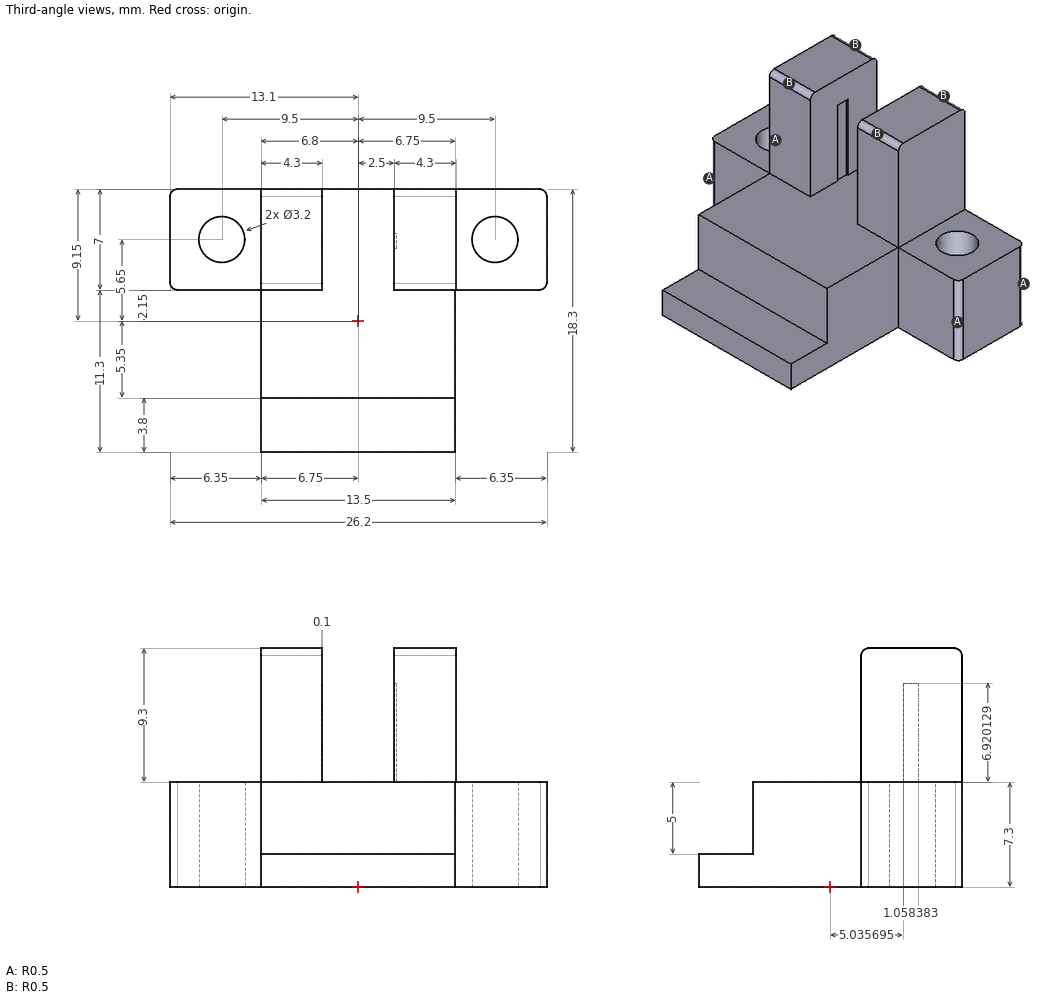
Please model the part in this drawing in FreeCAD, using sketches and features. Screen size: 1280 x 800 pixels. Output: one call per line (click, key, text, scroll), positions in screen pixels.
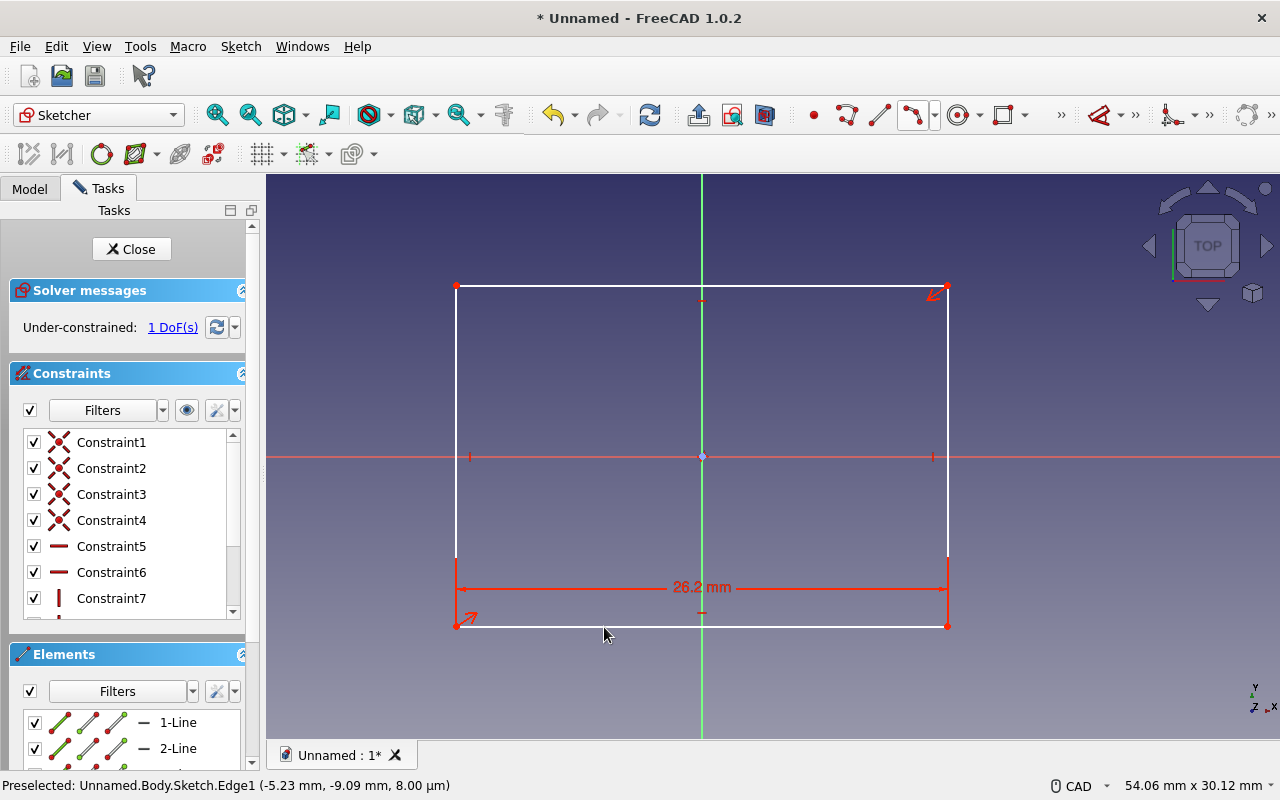
click(948, 525)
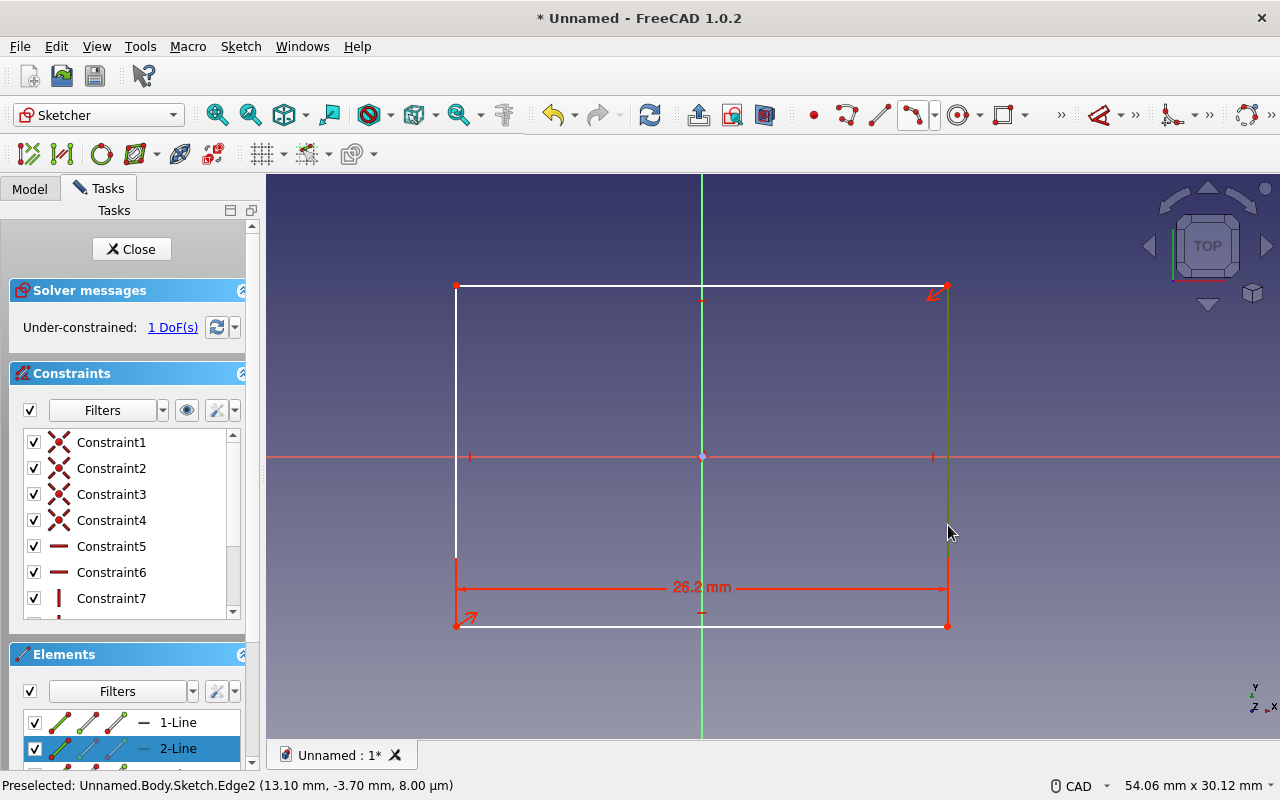
key(i)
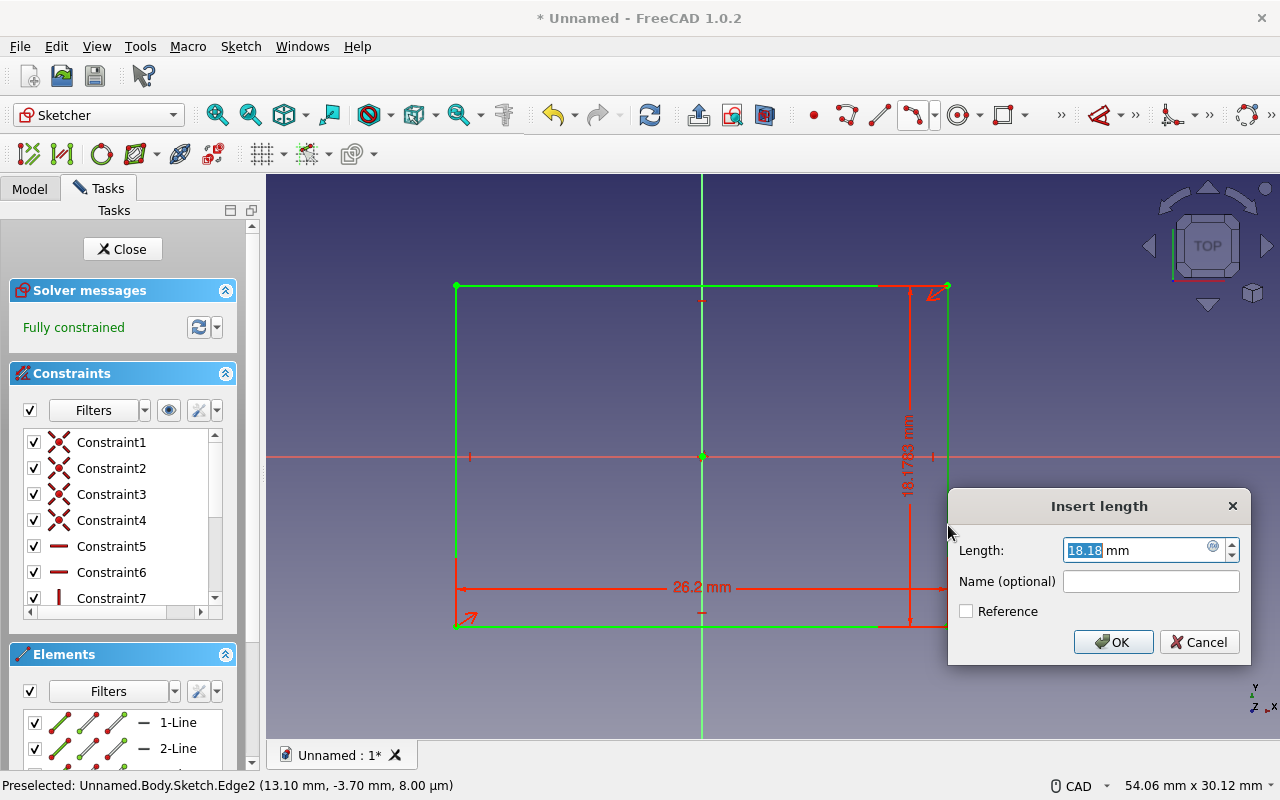
text(18.3)
key(Return)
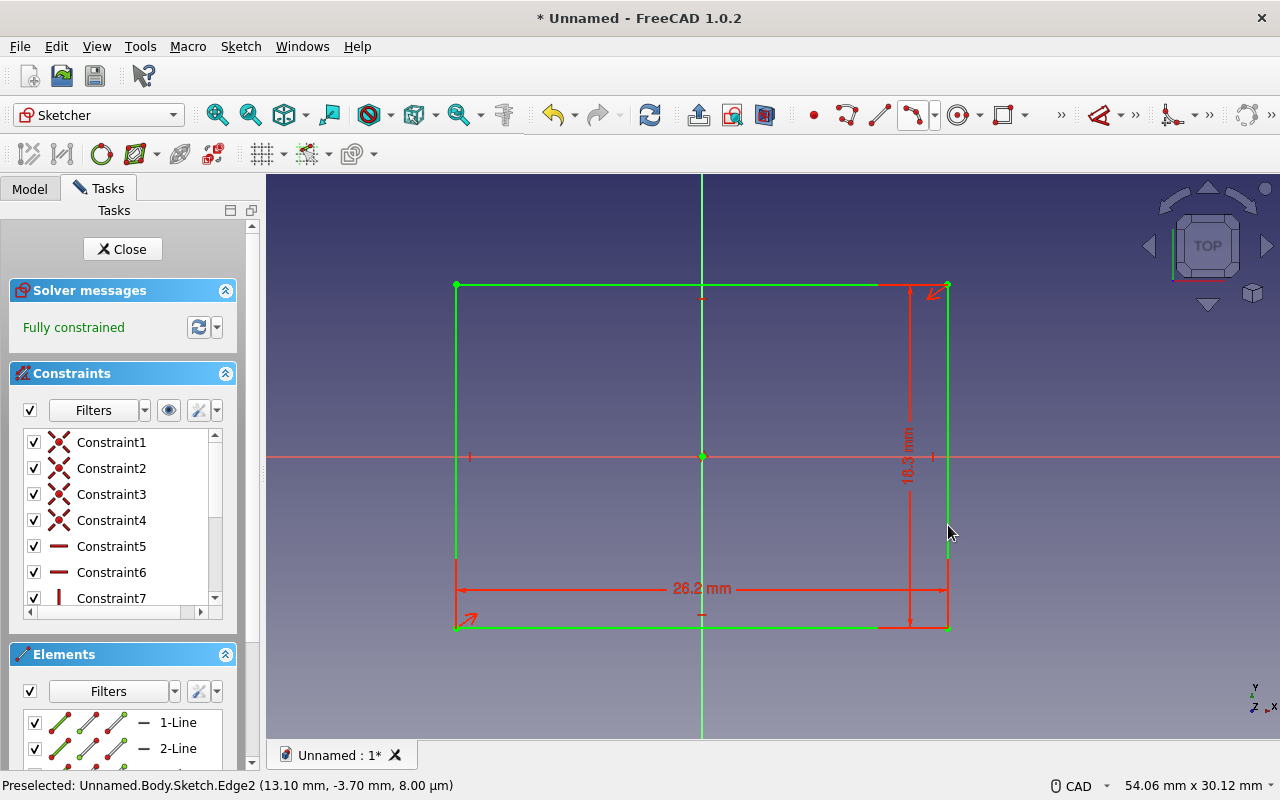
click(123, 249)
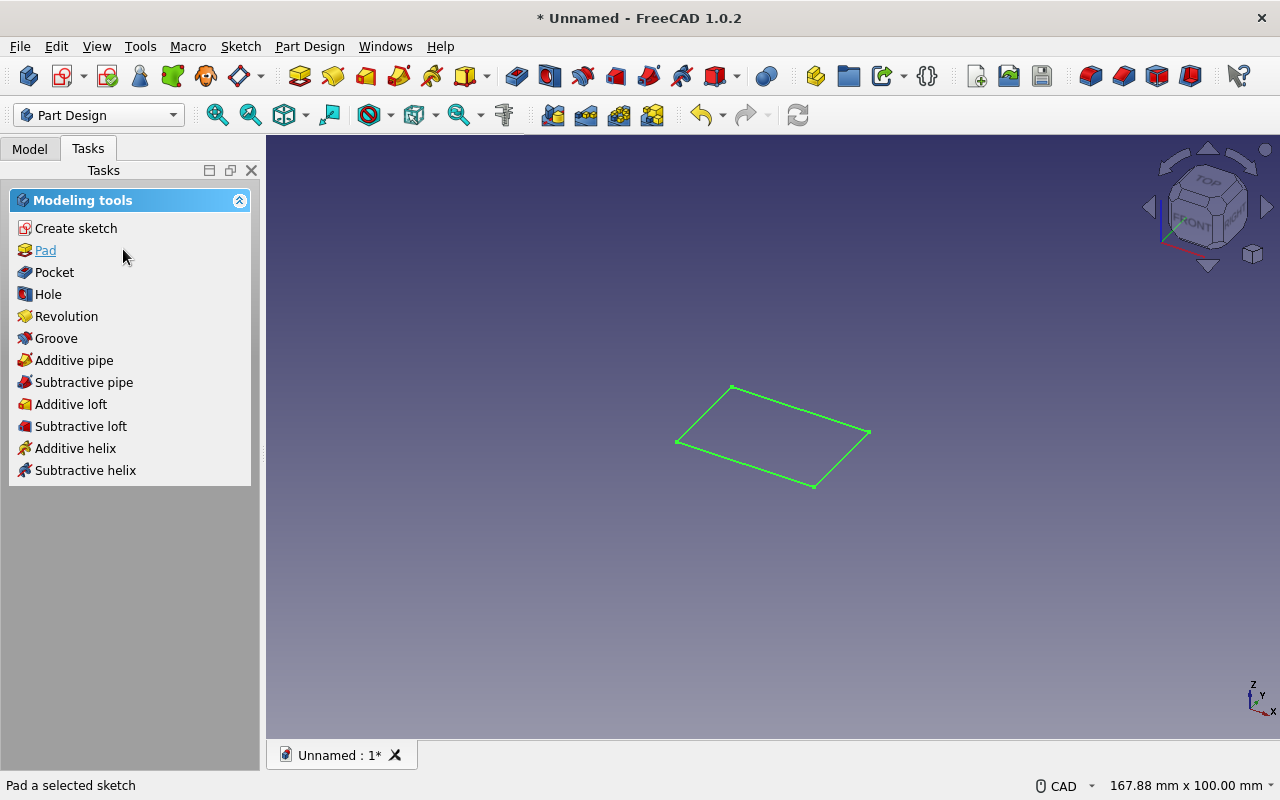
click(300, 76)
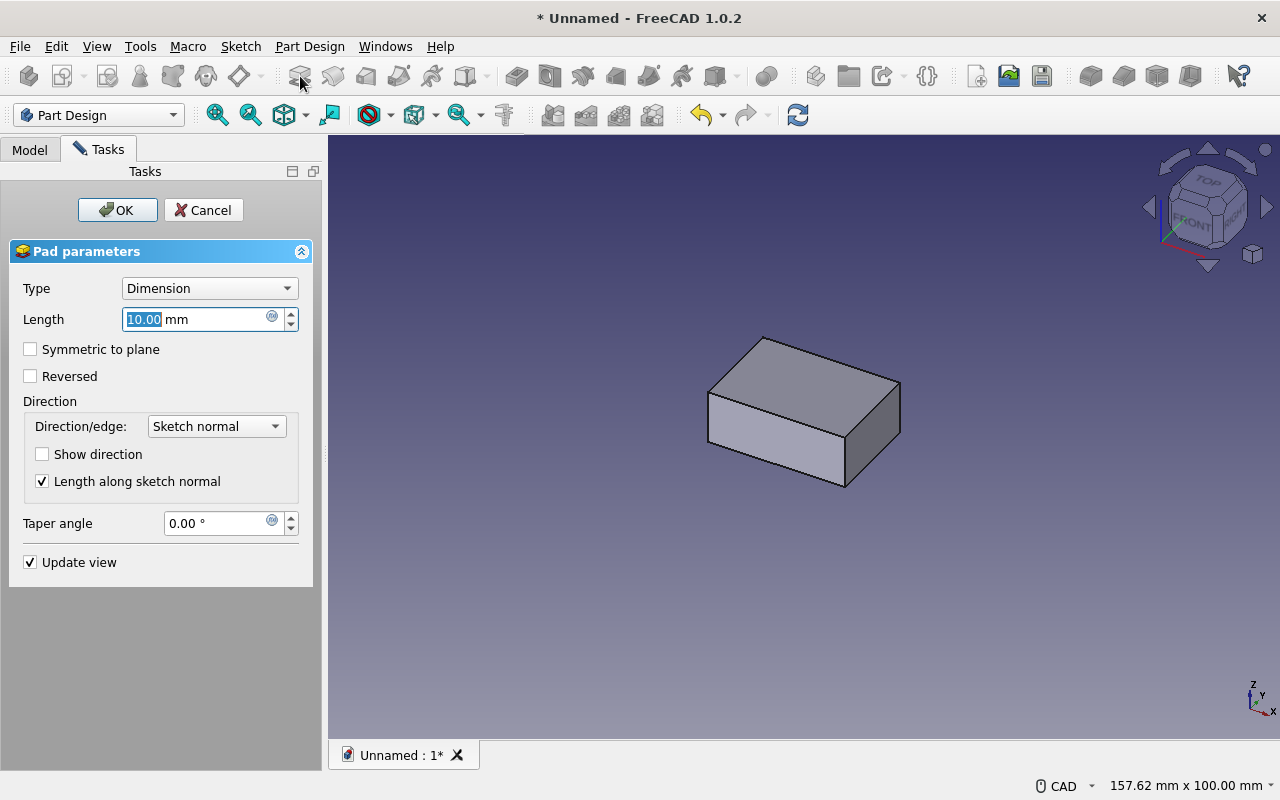
text(7.3)
key(Tab)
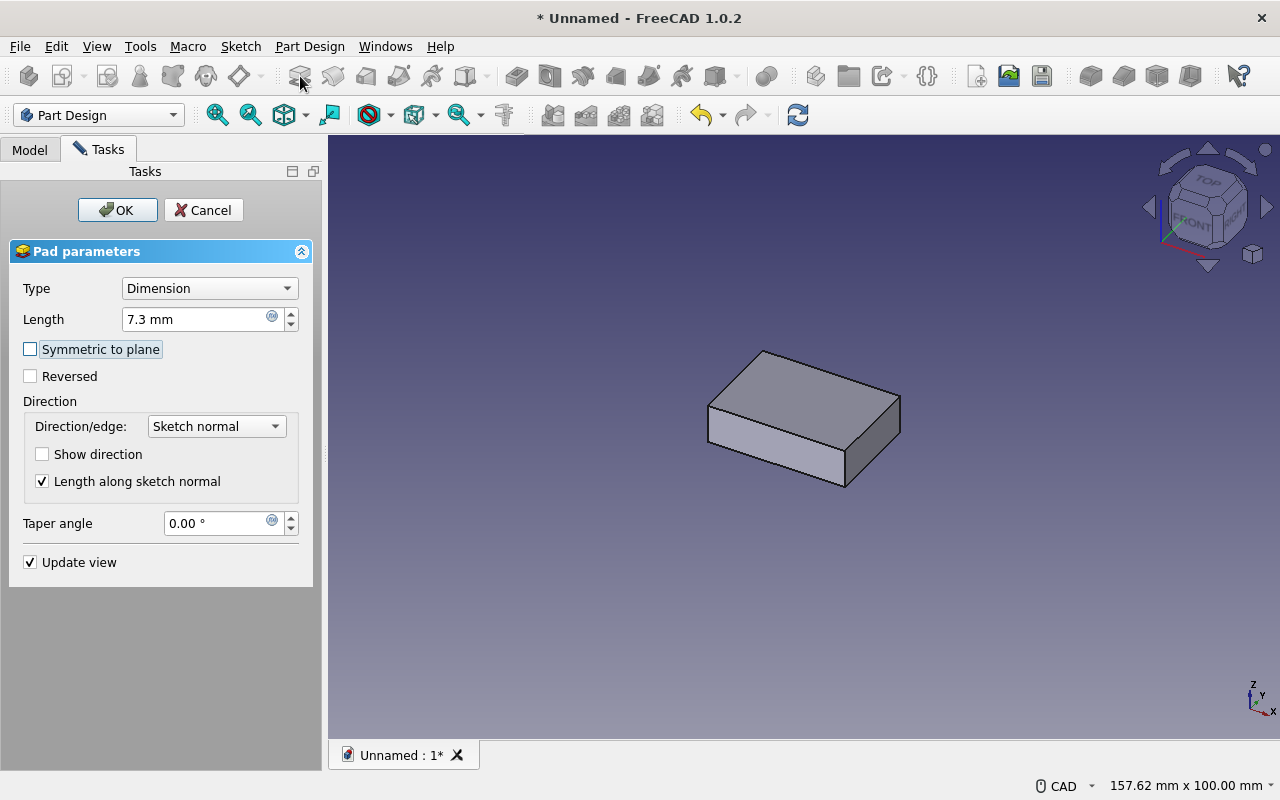
click(118, 210)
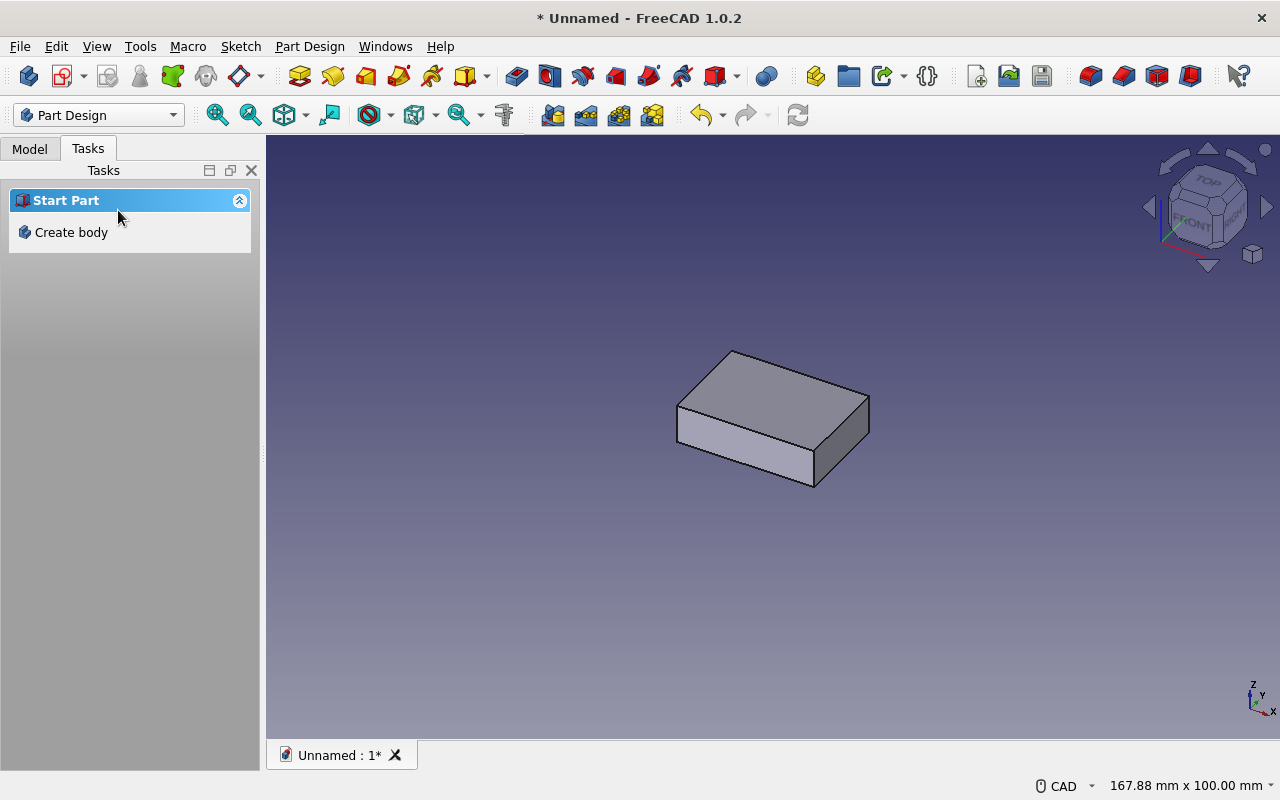
click(218, 116)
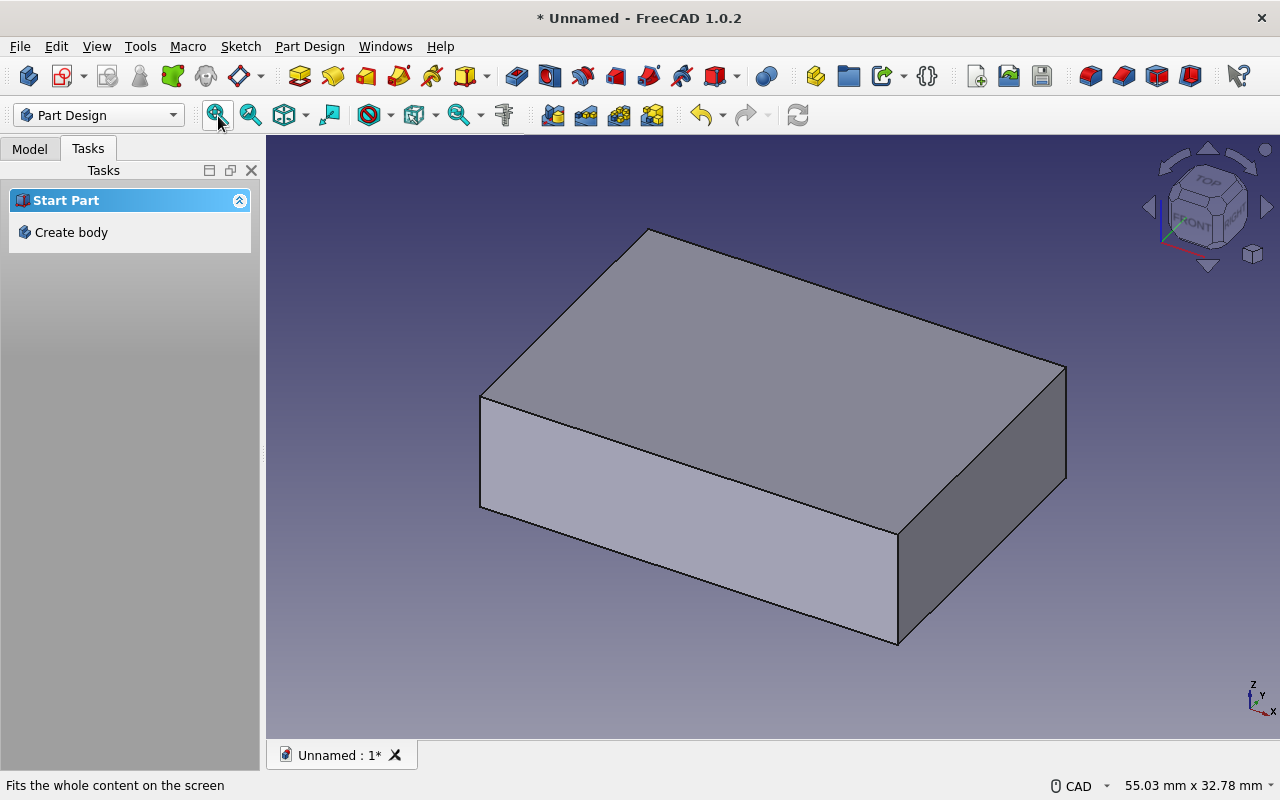
click(833, 401)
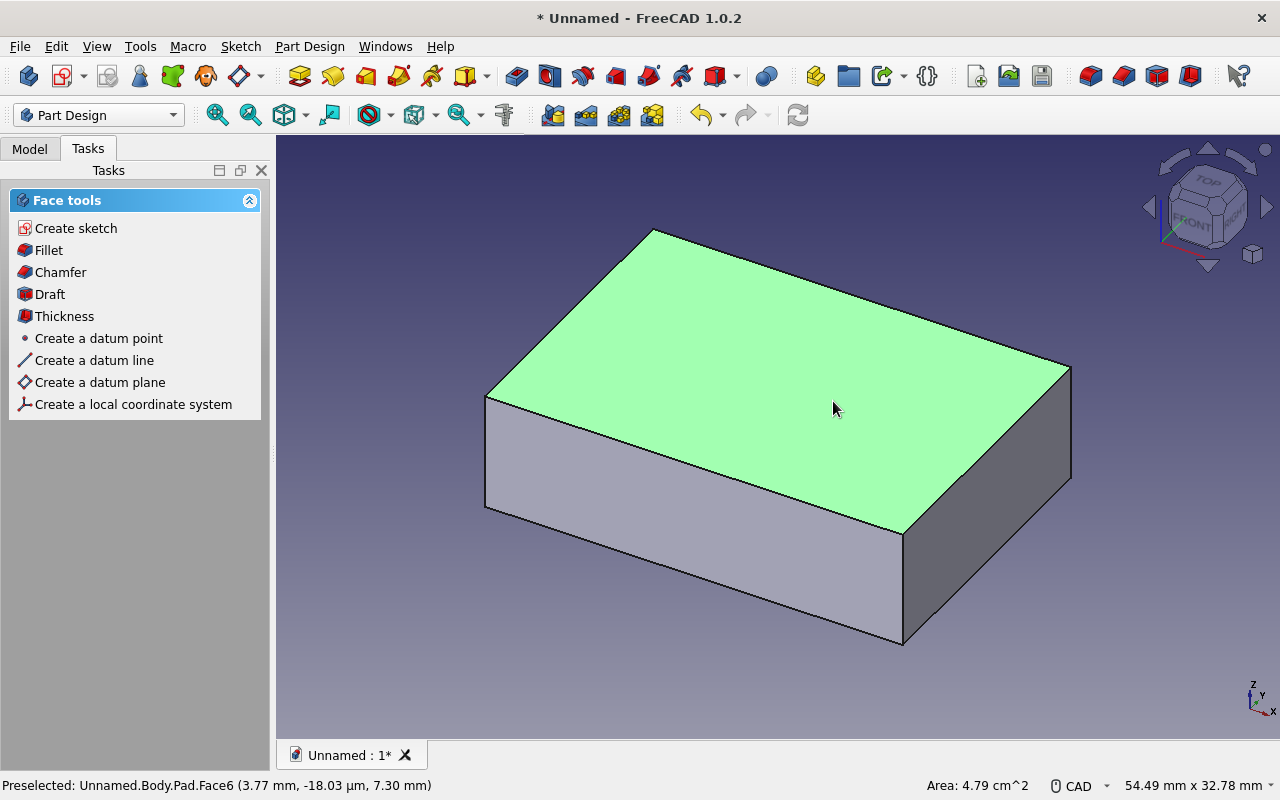
click(62, 76)